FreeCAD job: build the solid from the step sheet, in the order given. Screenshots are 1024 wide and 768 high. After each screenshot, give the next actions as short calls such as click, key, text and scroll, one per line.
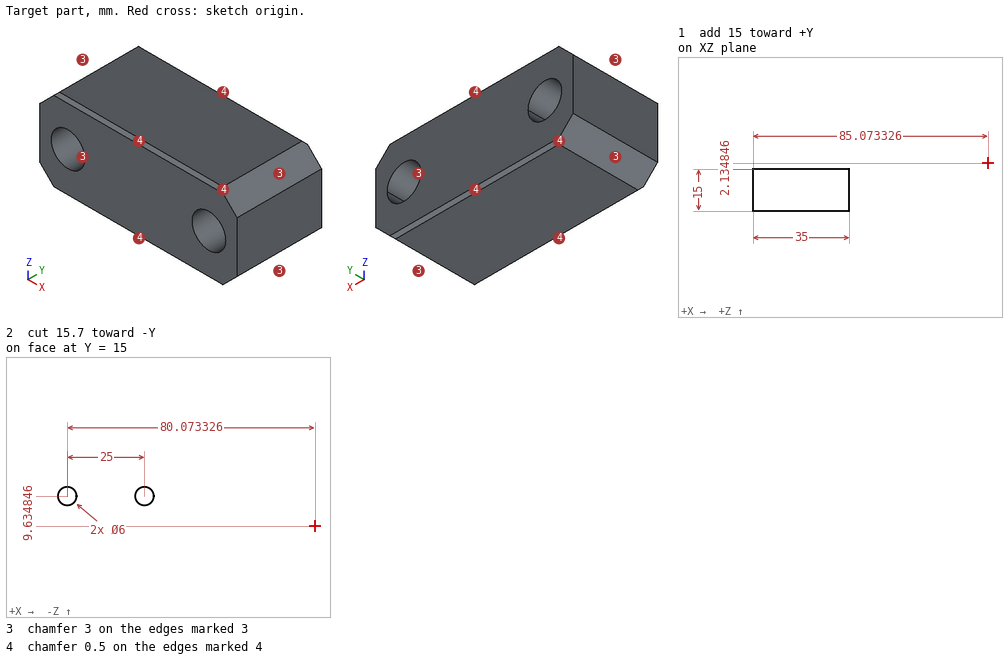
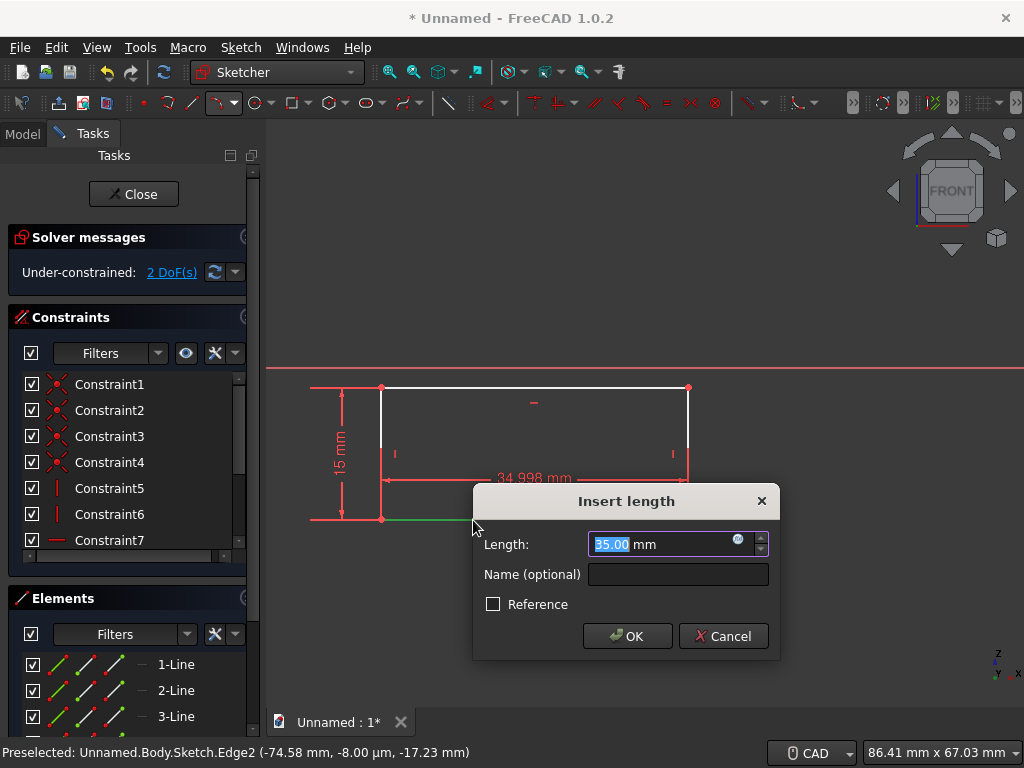
text(35)
key(Return)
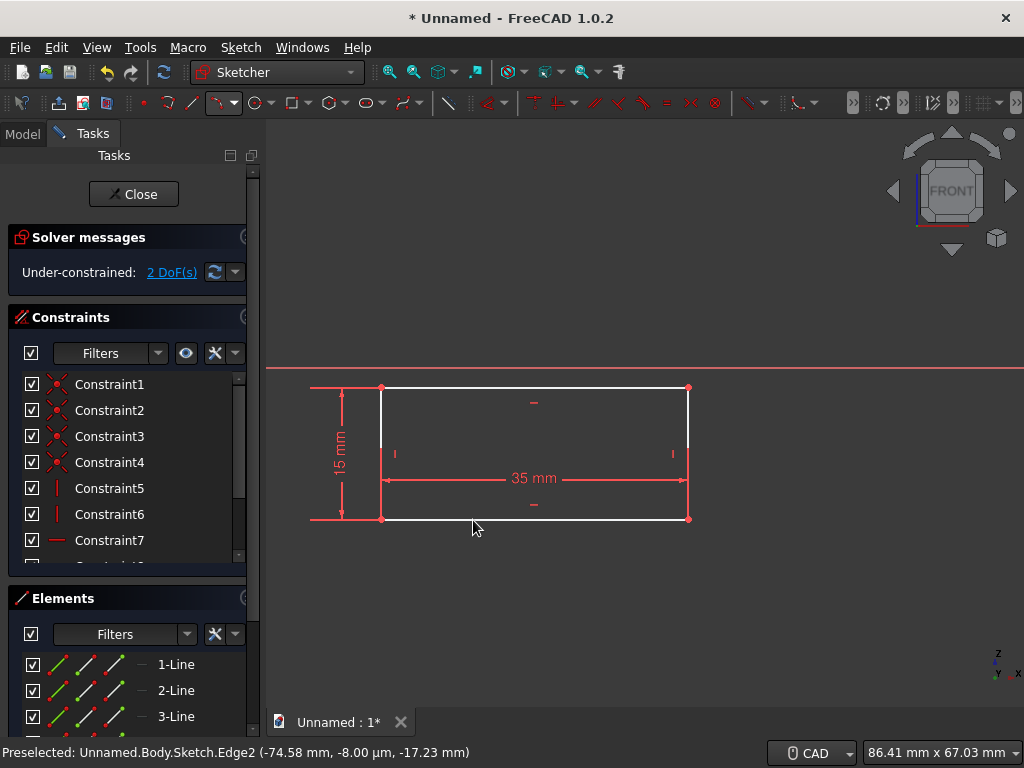
scroll(381, 388, up, 4)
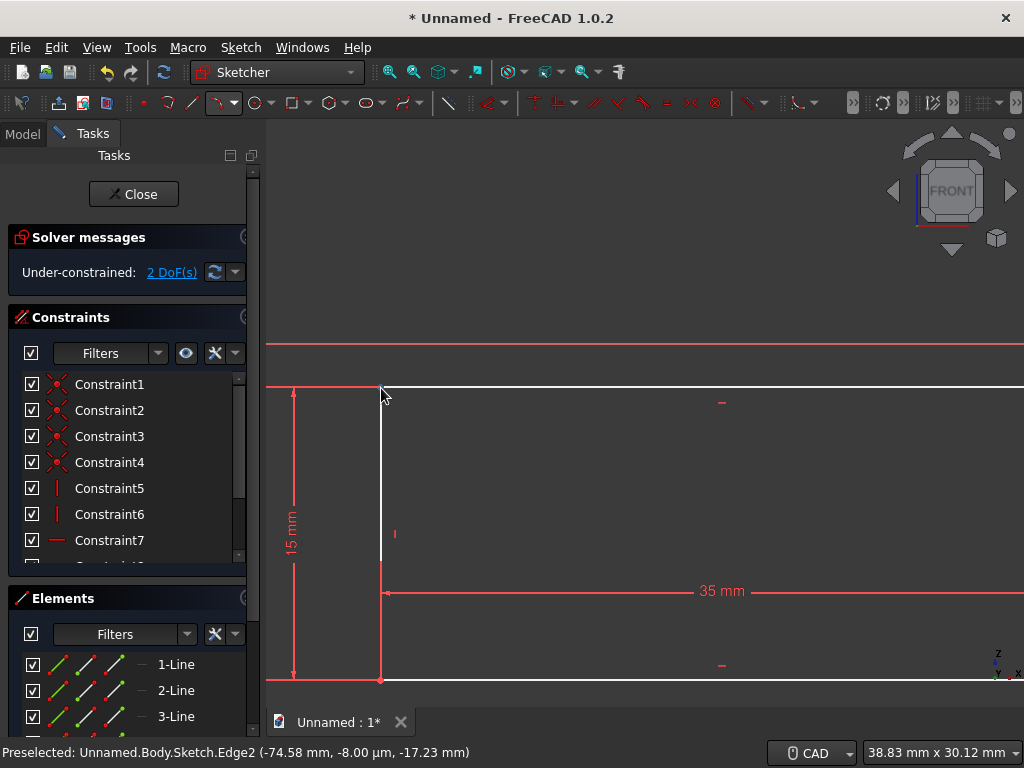
click(381, 387)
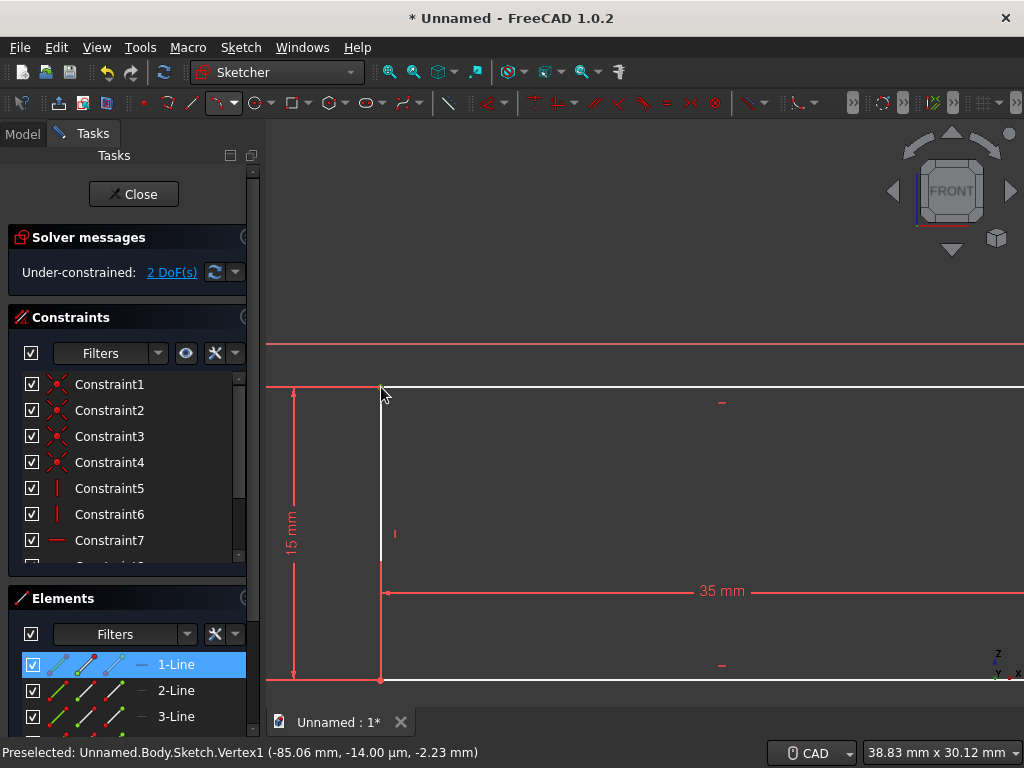
key(i)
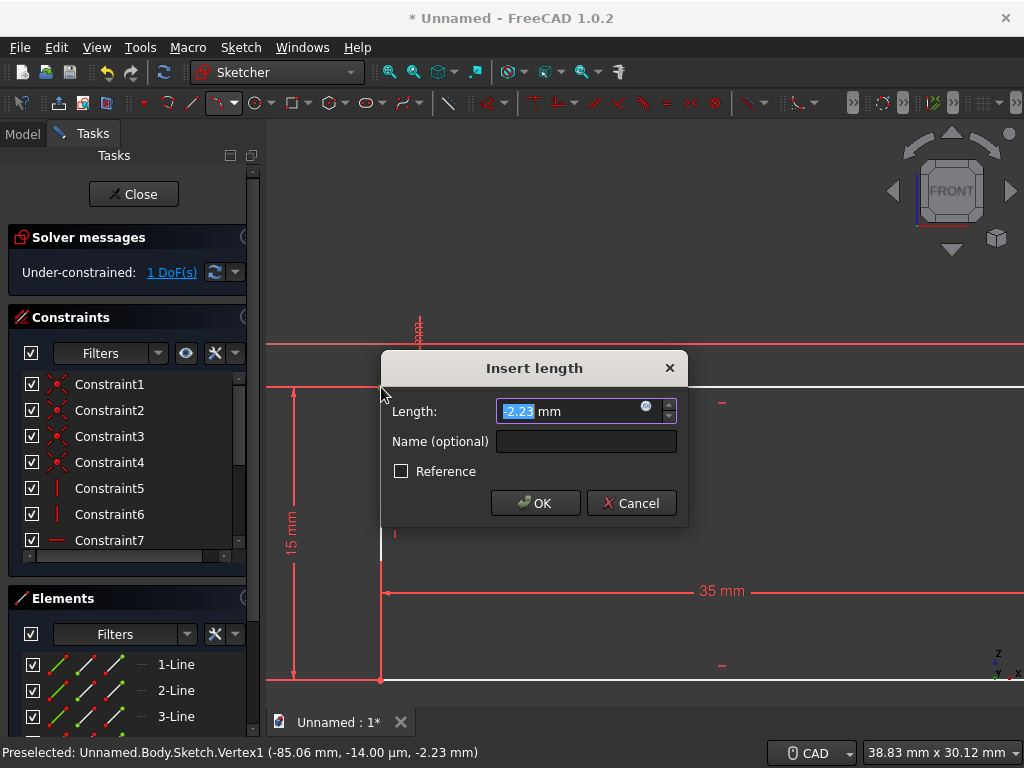
text(-2.134846)
key(Return)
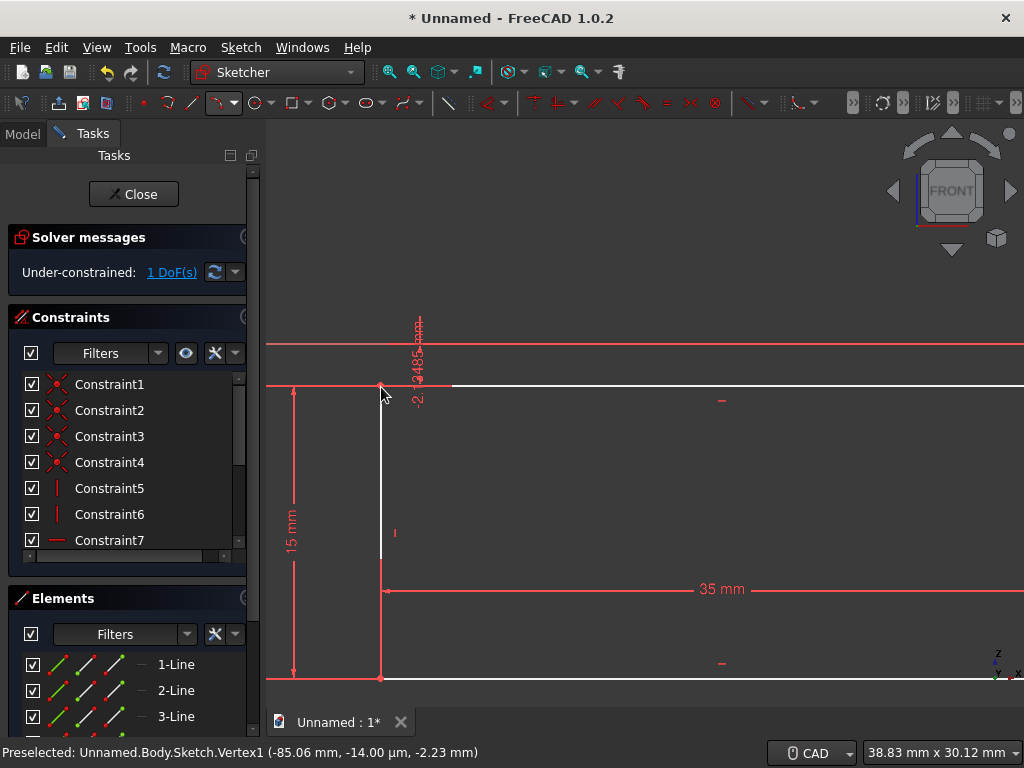
scroll(369, 381, down, 7)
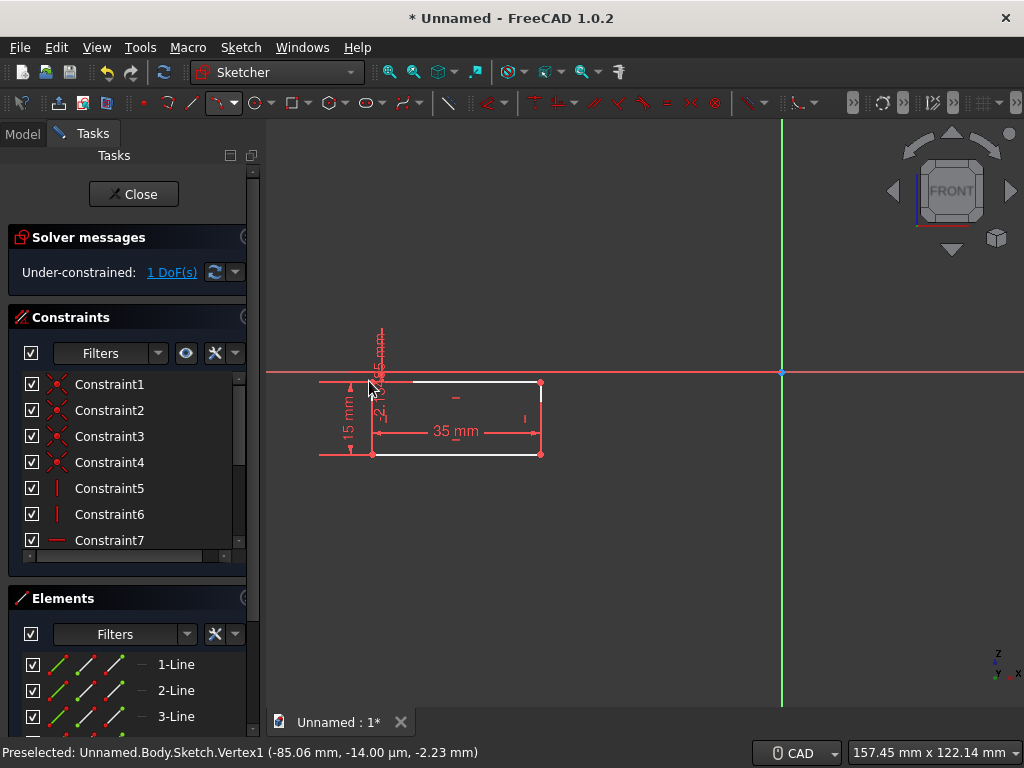
click(372, 382)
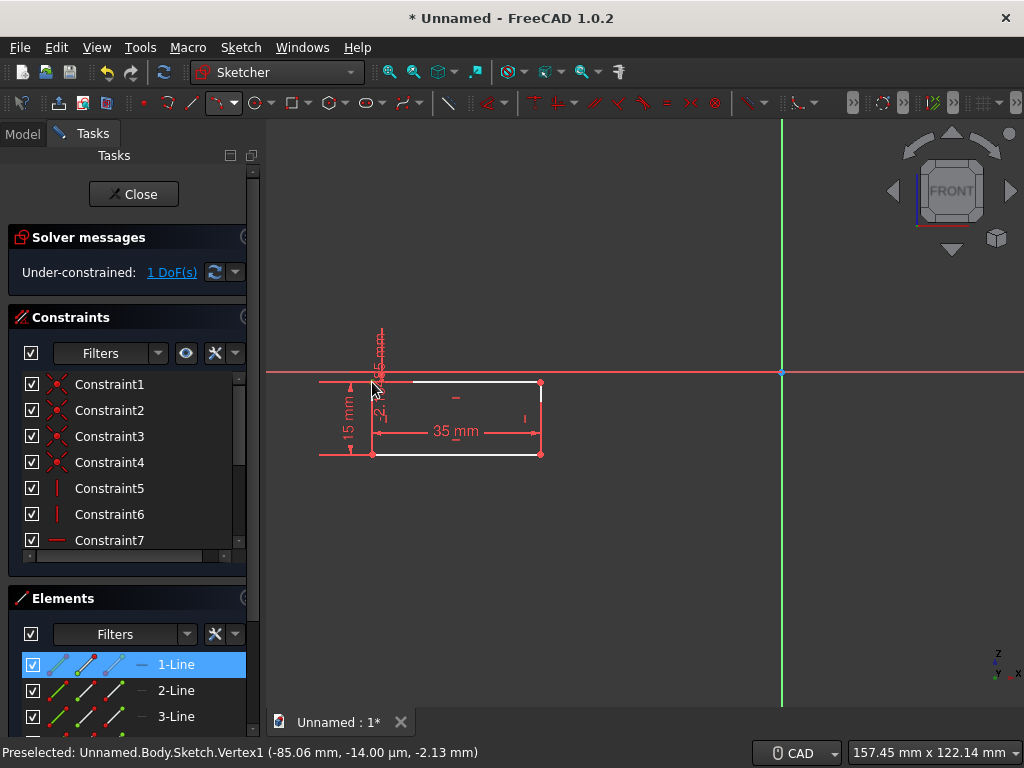
key(l)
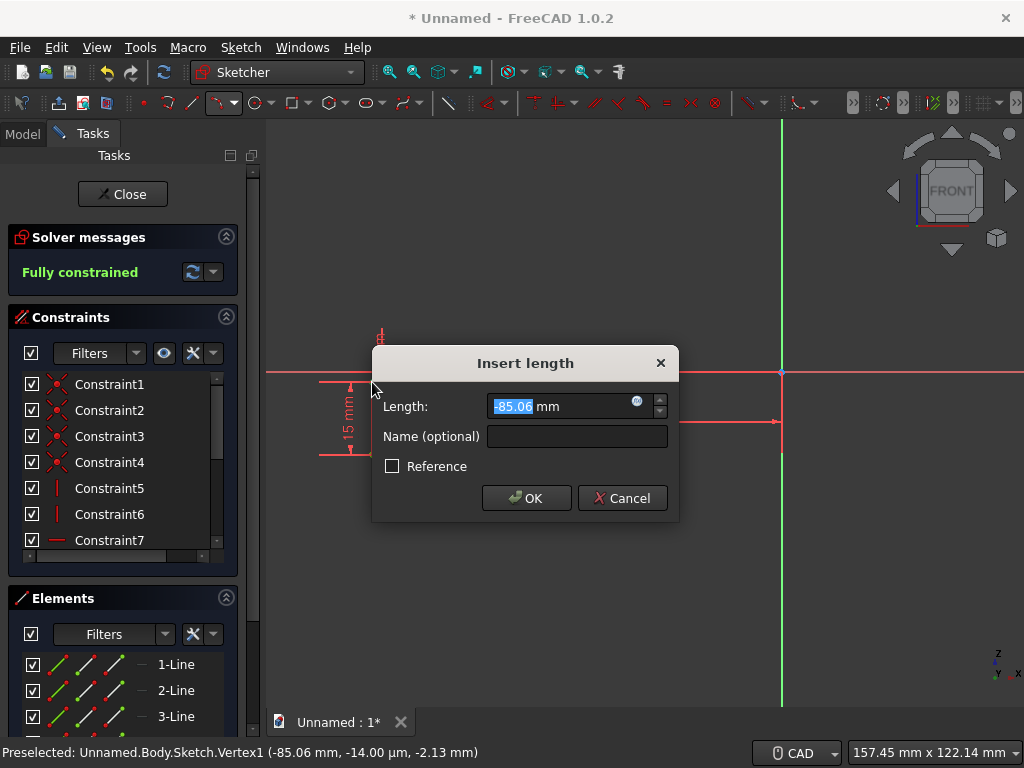
text(-85.073326)
key(Return)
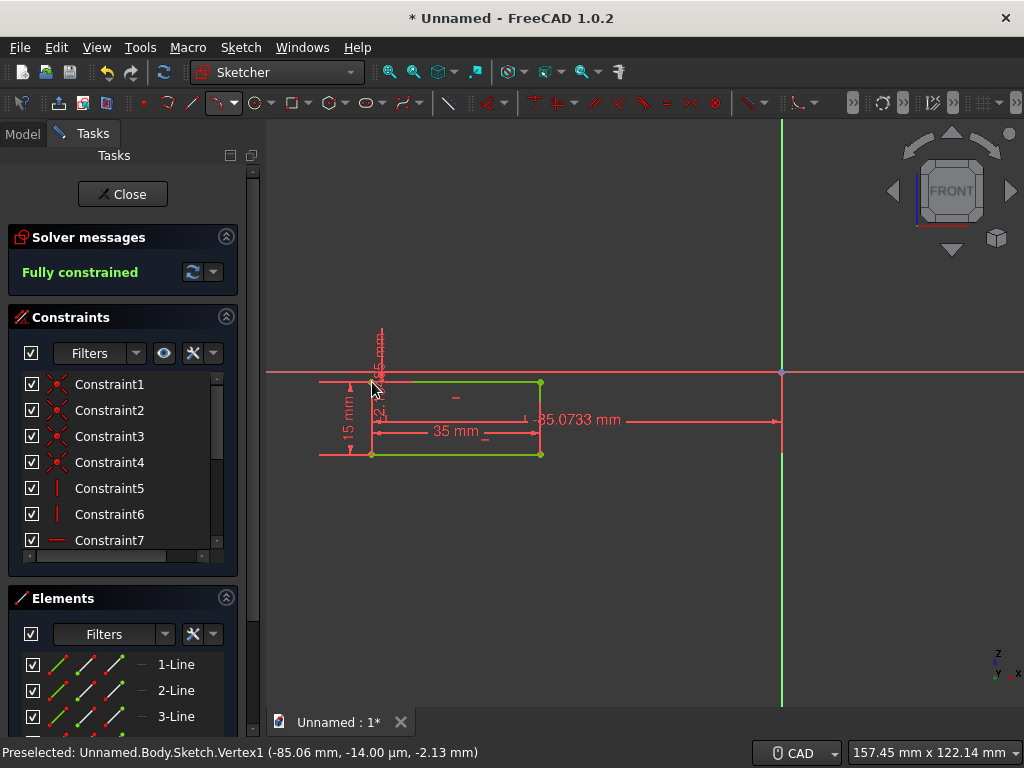
click(123, 194)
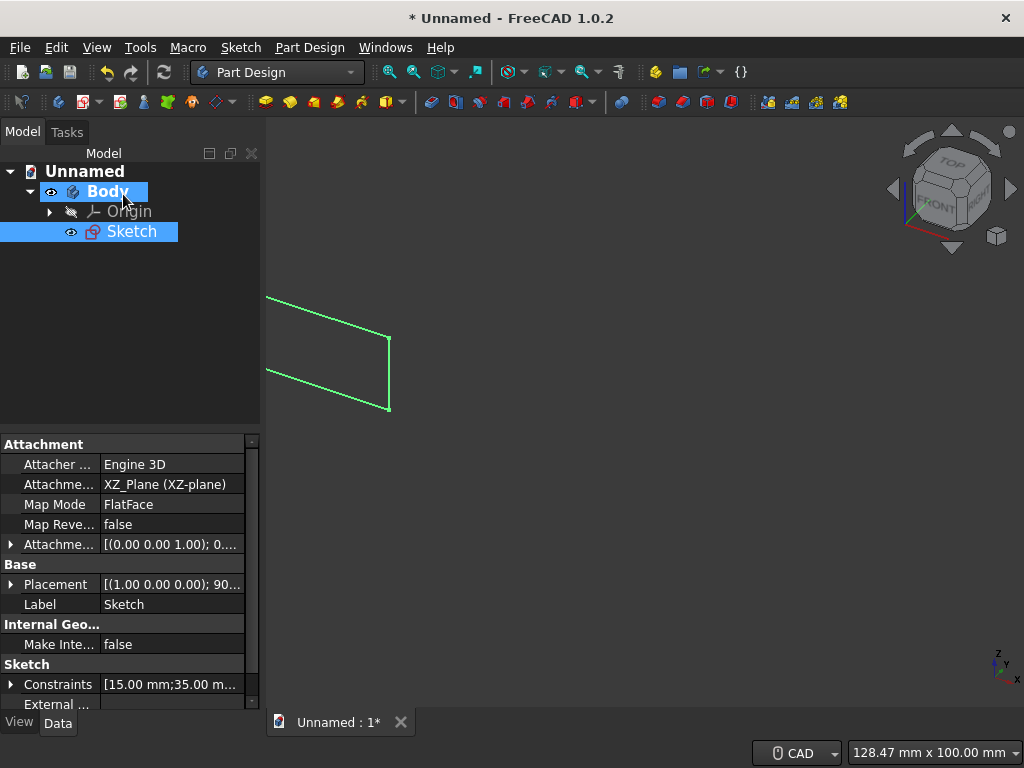
click(266, 102)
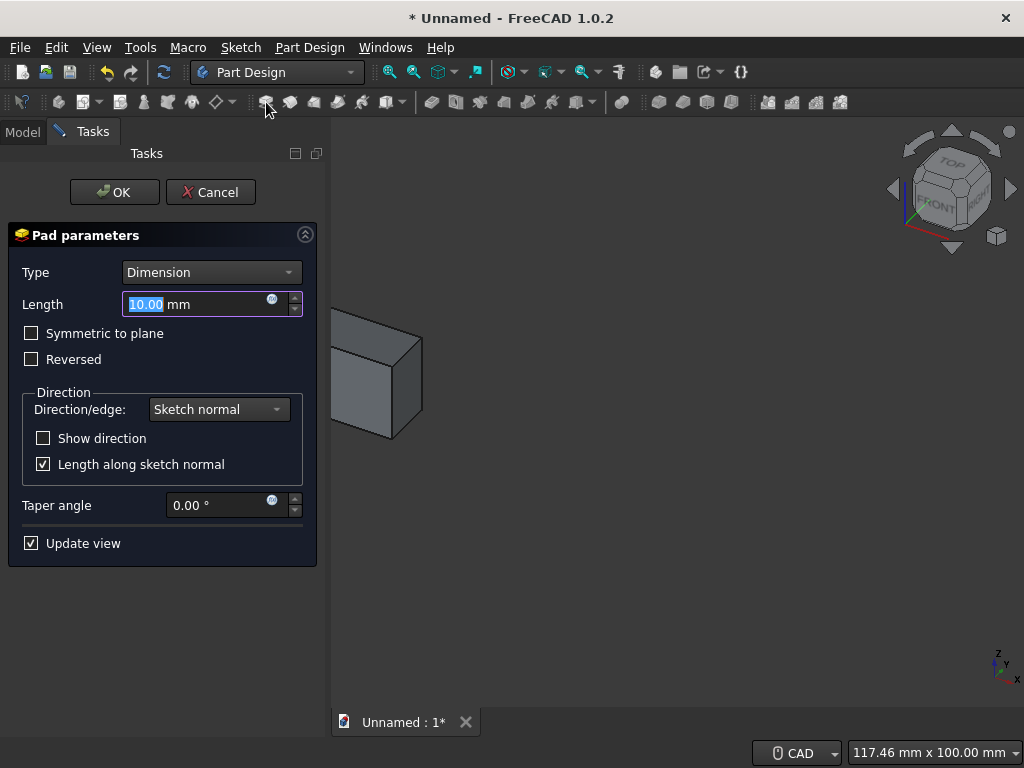
text(15)
key(Tab)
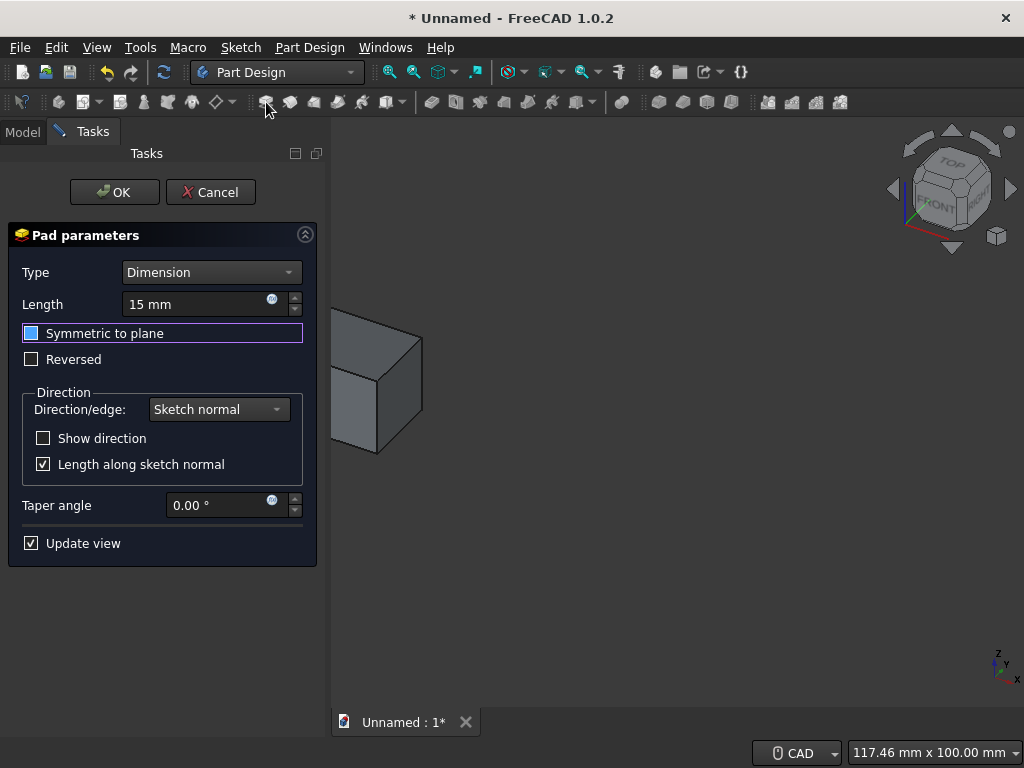
click(30, 359)